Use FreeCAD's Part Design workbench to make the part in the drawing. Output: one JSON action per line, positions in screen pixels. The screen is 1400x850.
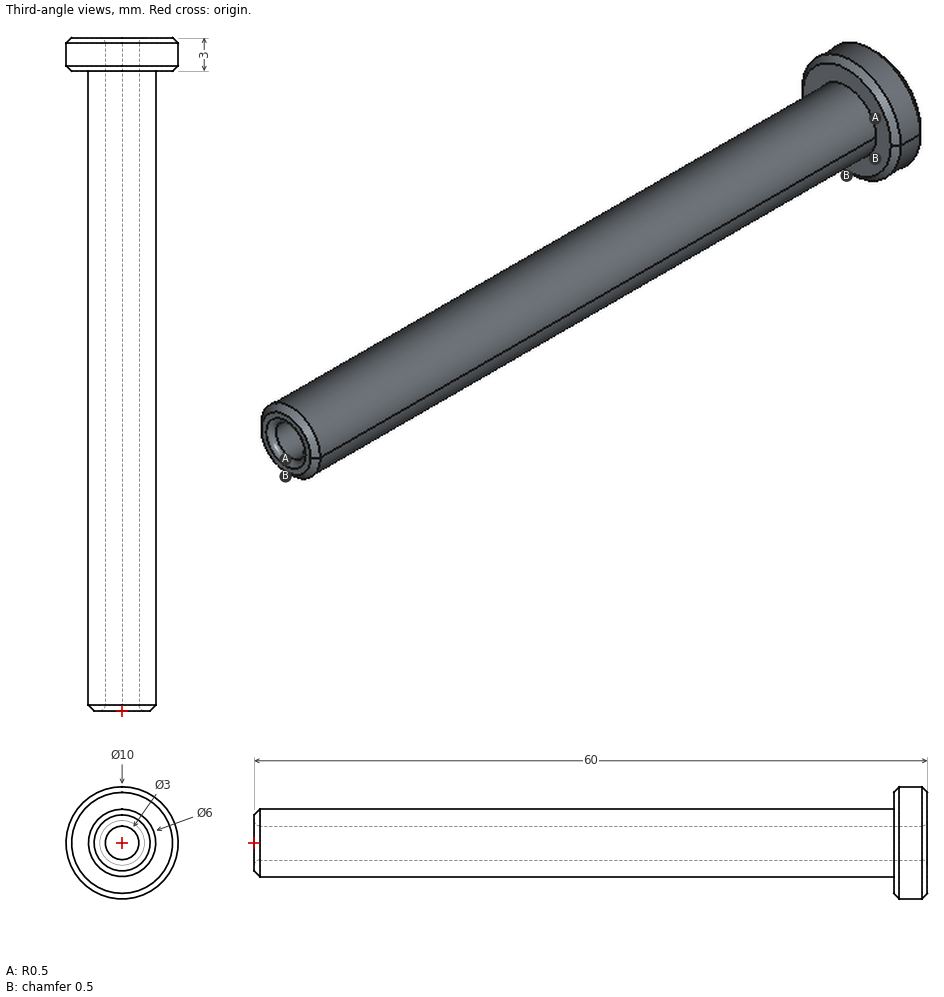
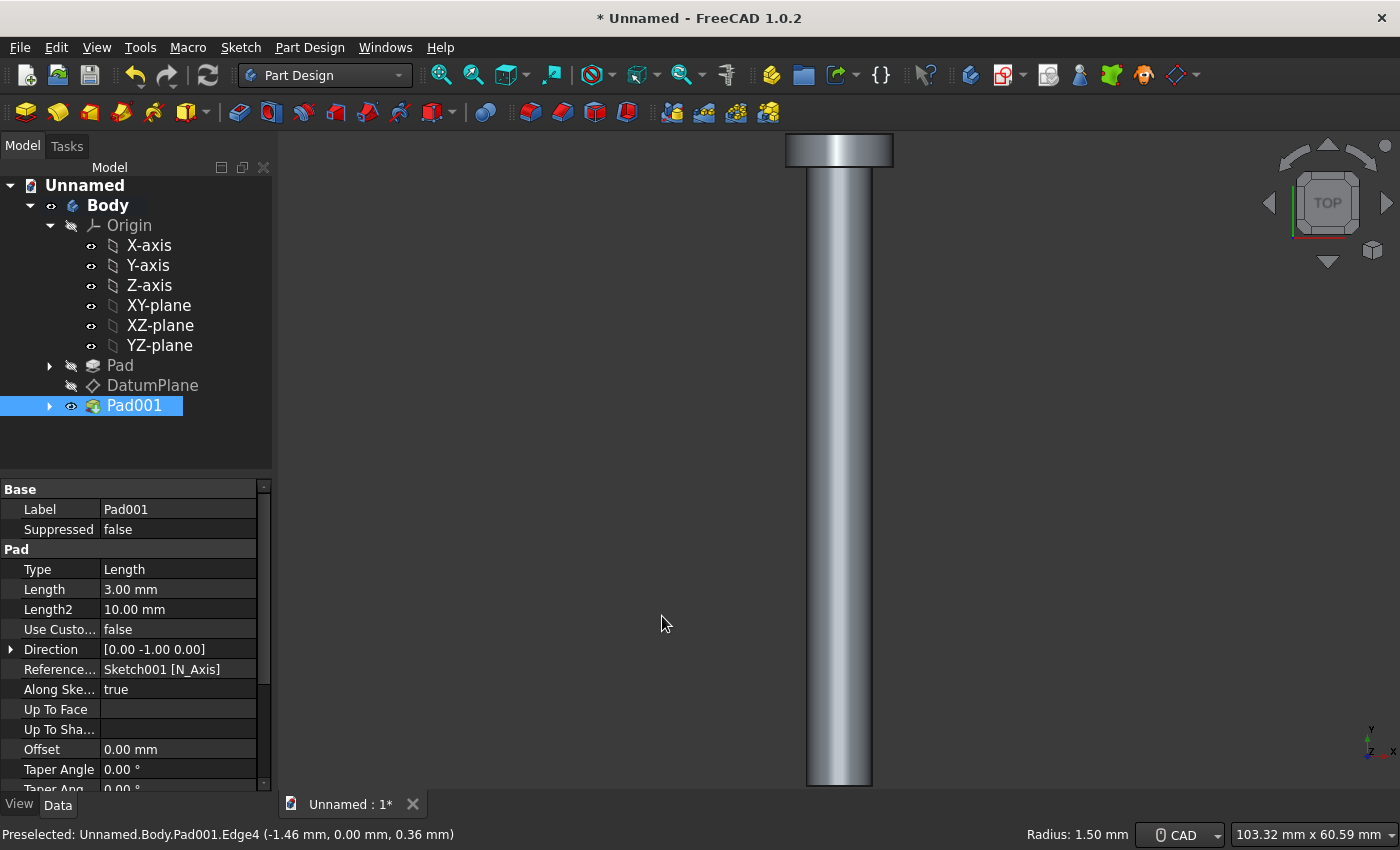
{"action": "key", "text": "1"}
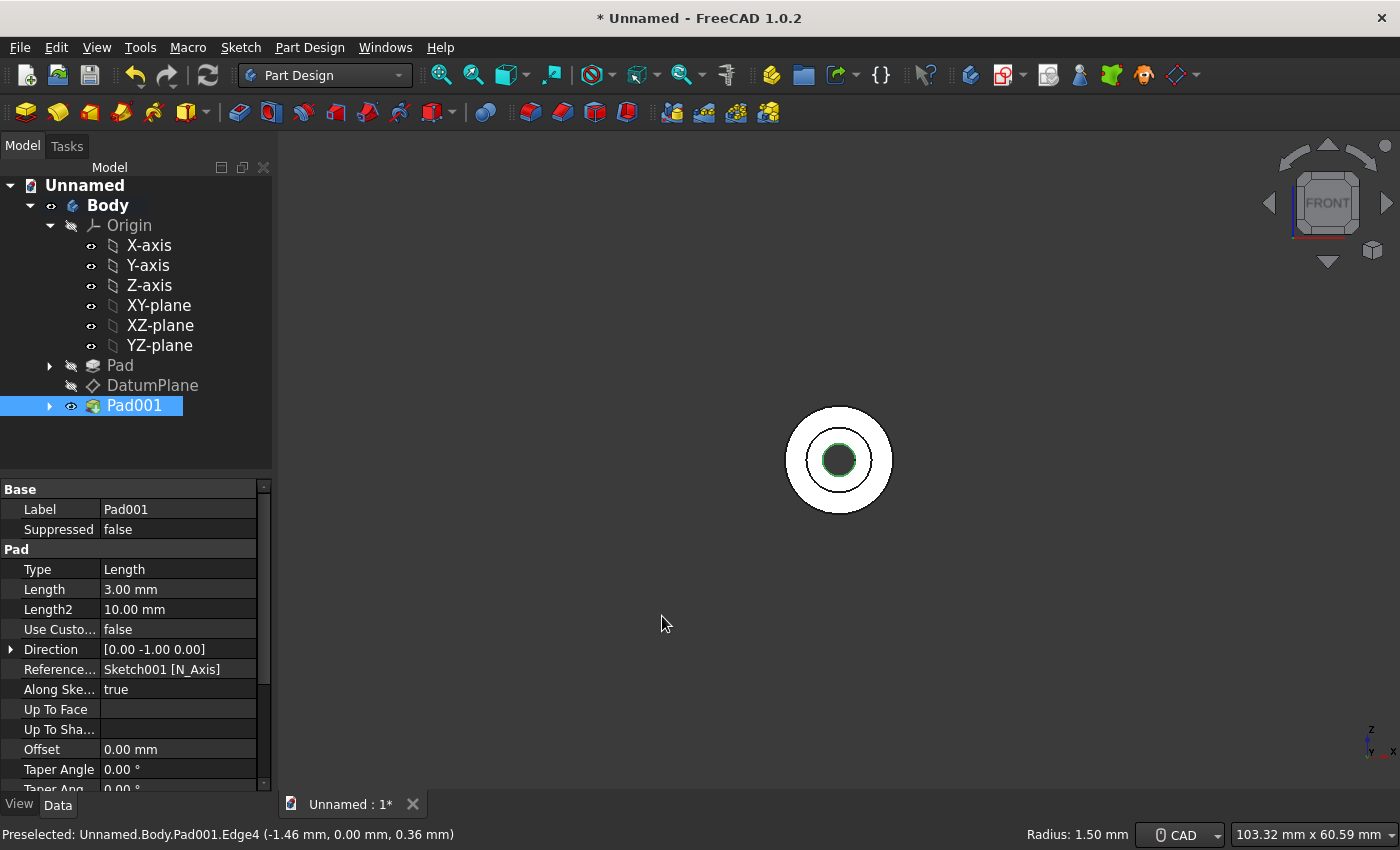
{"action": "key", "text": "v f"}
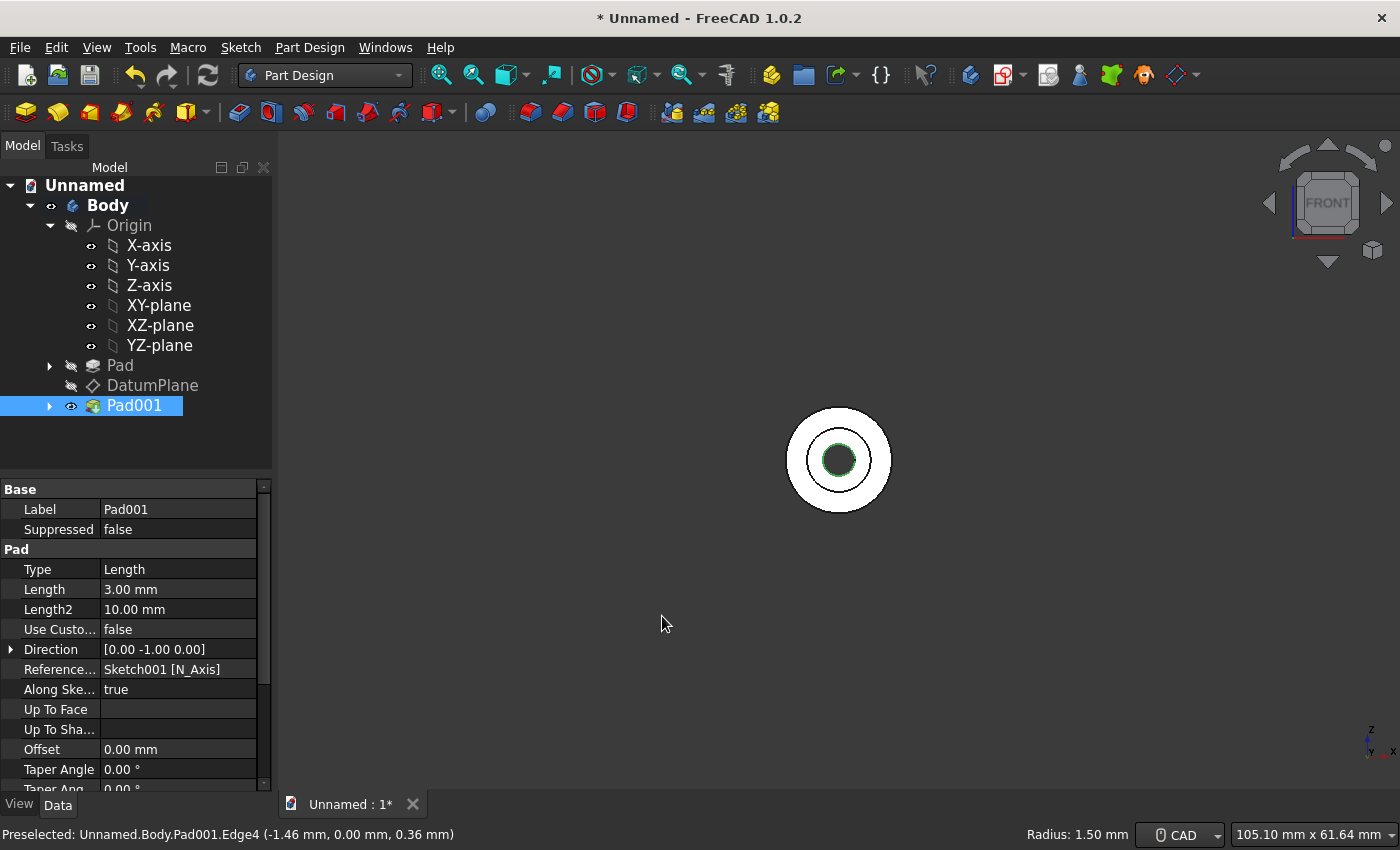
{"action": "key", "text": "3"}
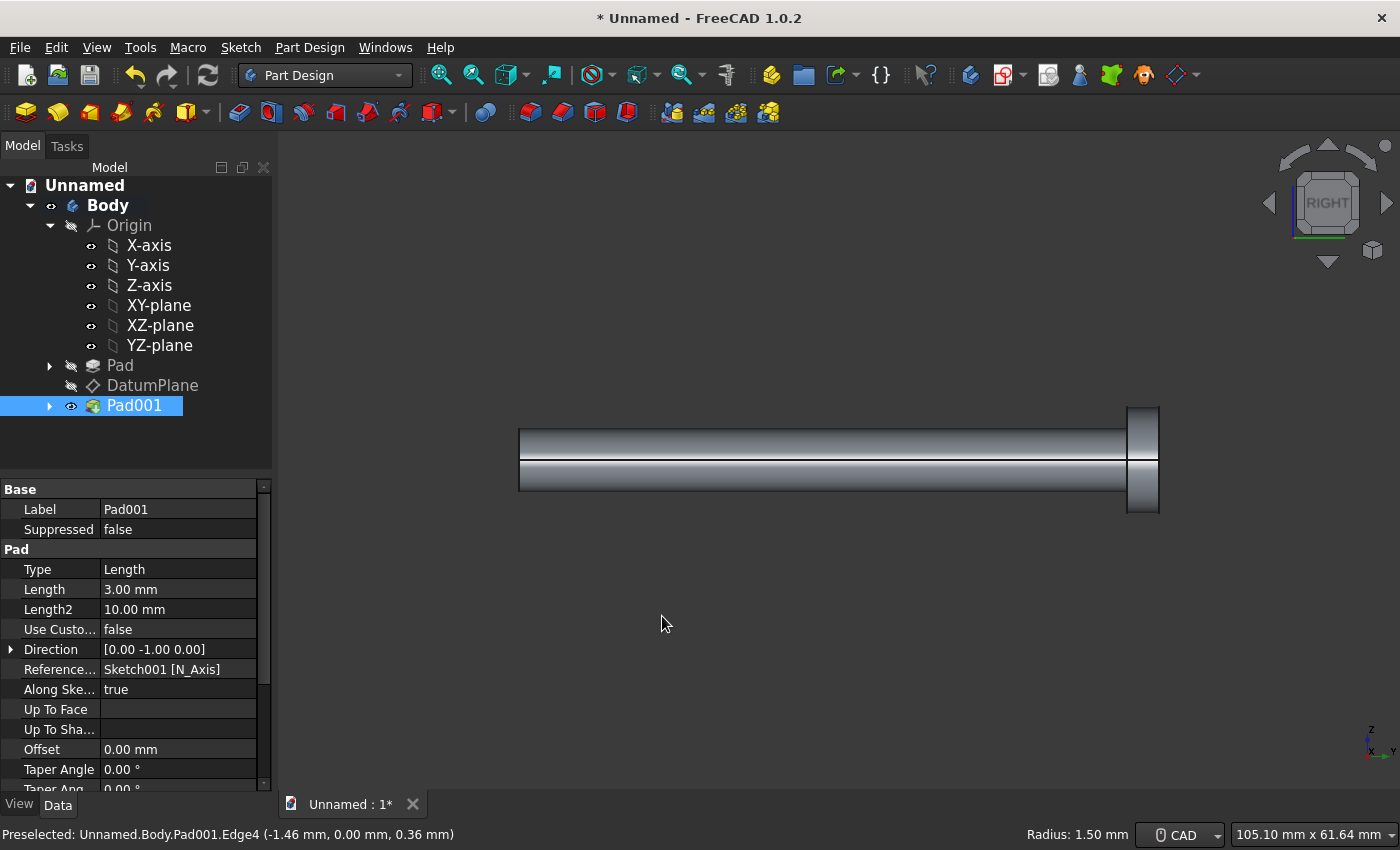
{"action": "key", "text": "5"}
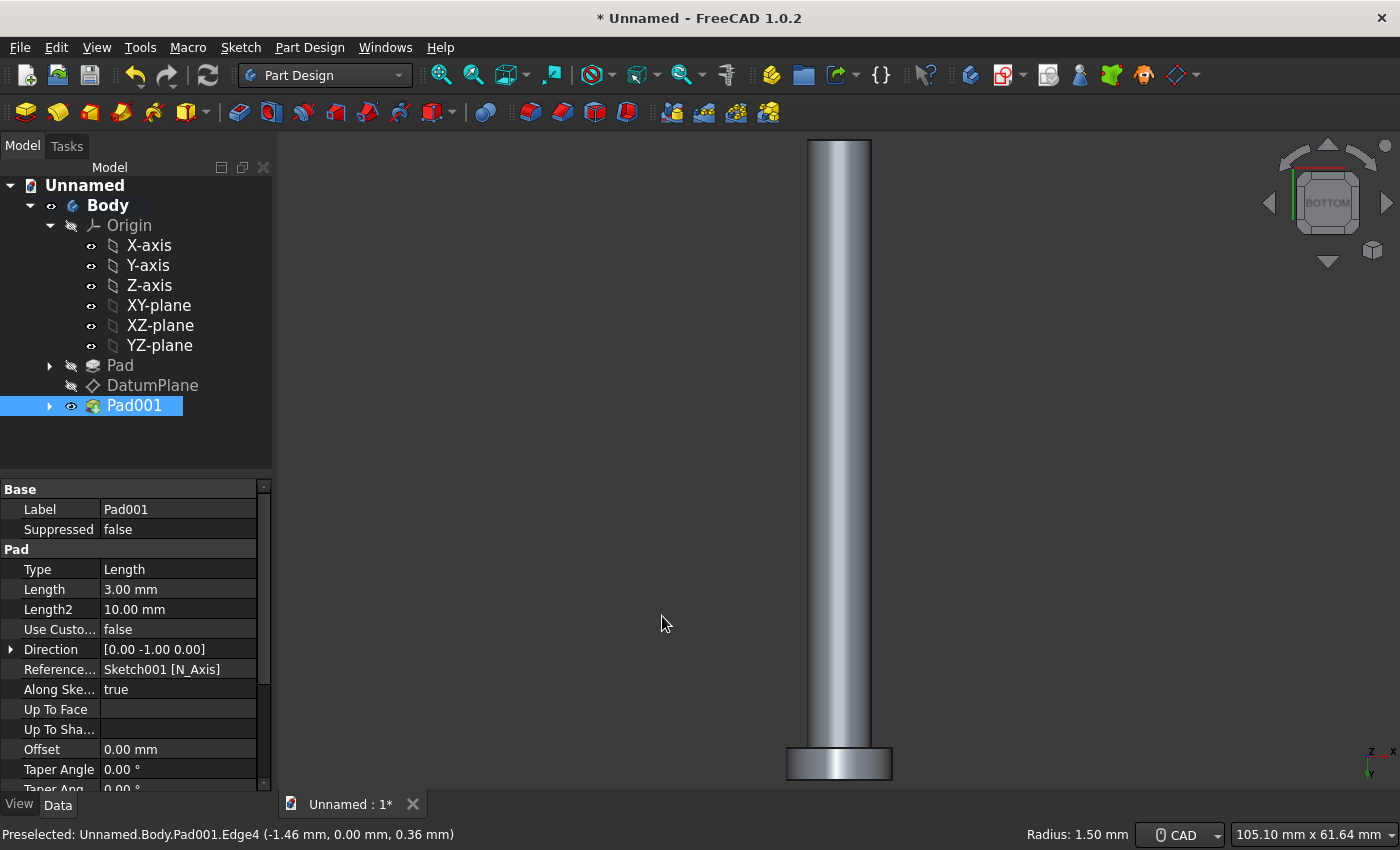
{"action": "key", "text": "4"}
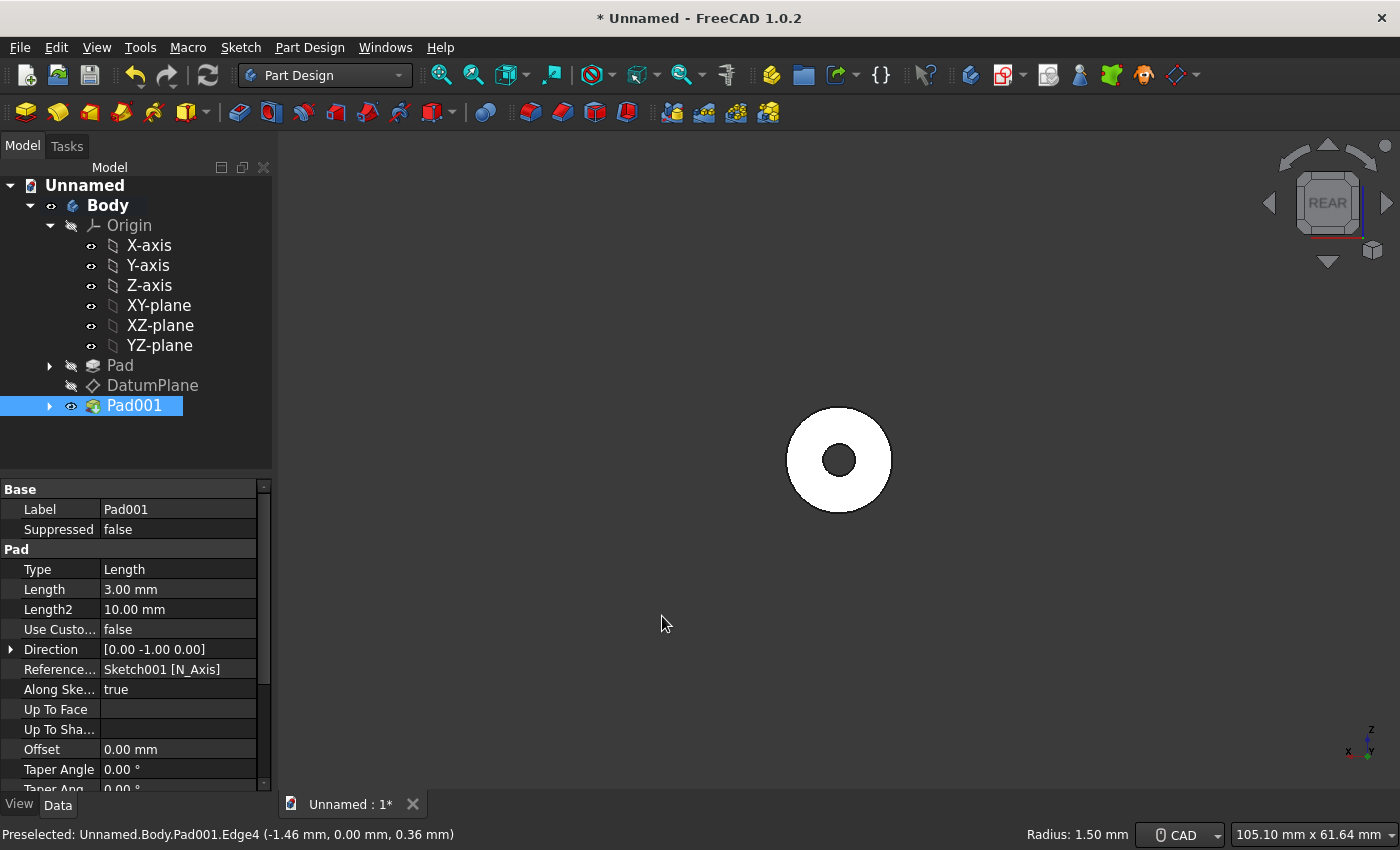
{"action": "left_click", "coordinate": [442, 76]}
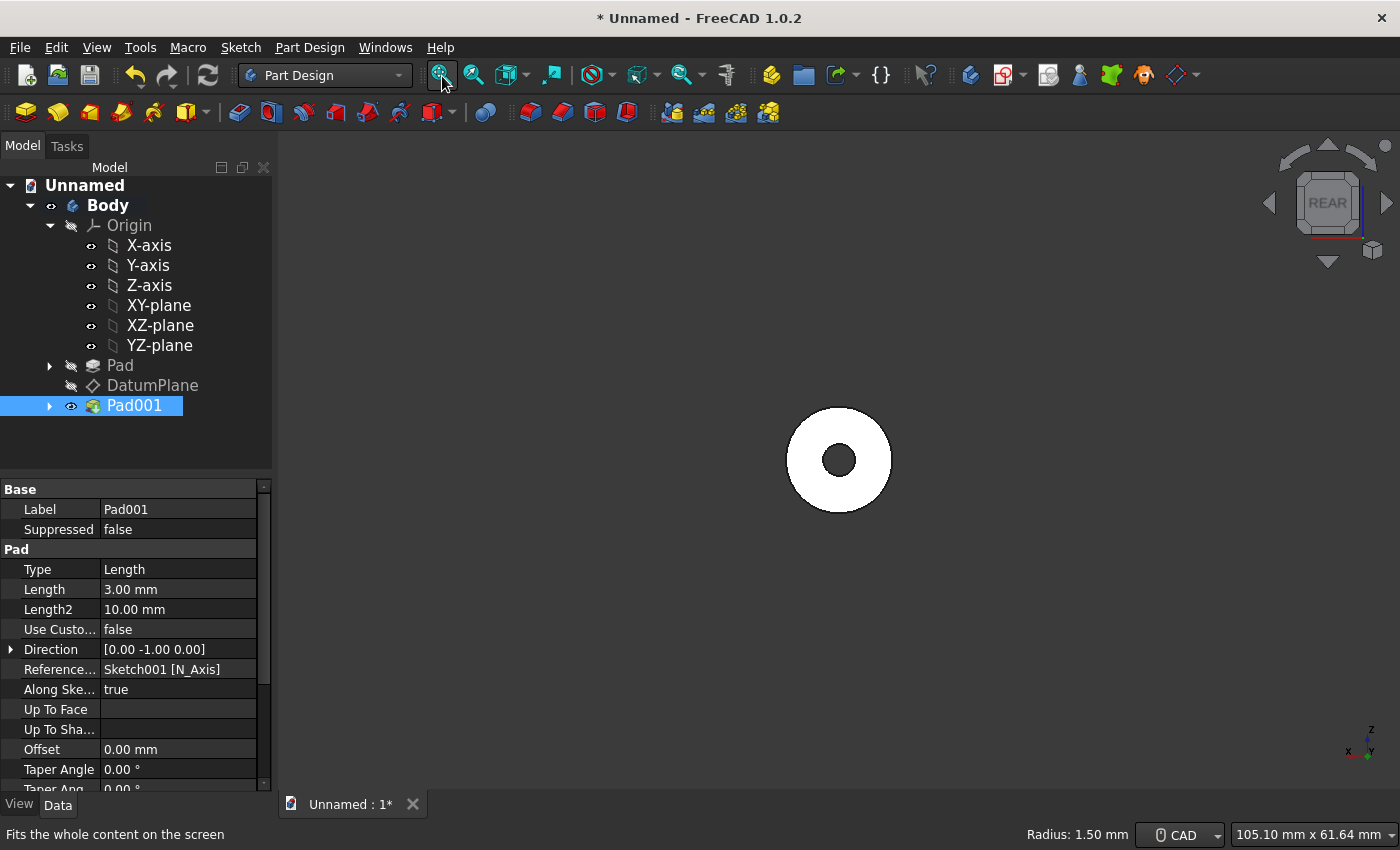
{"action": "left_click", "coordinate": [855, 459], "text": "ctrl"}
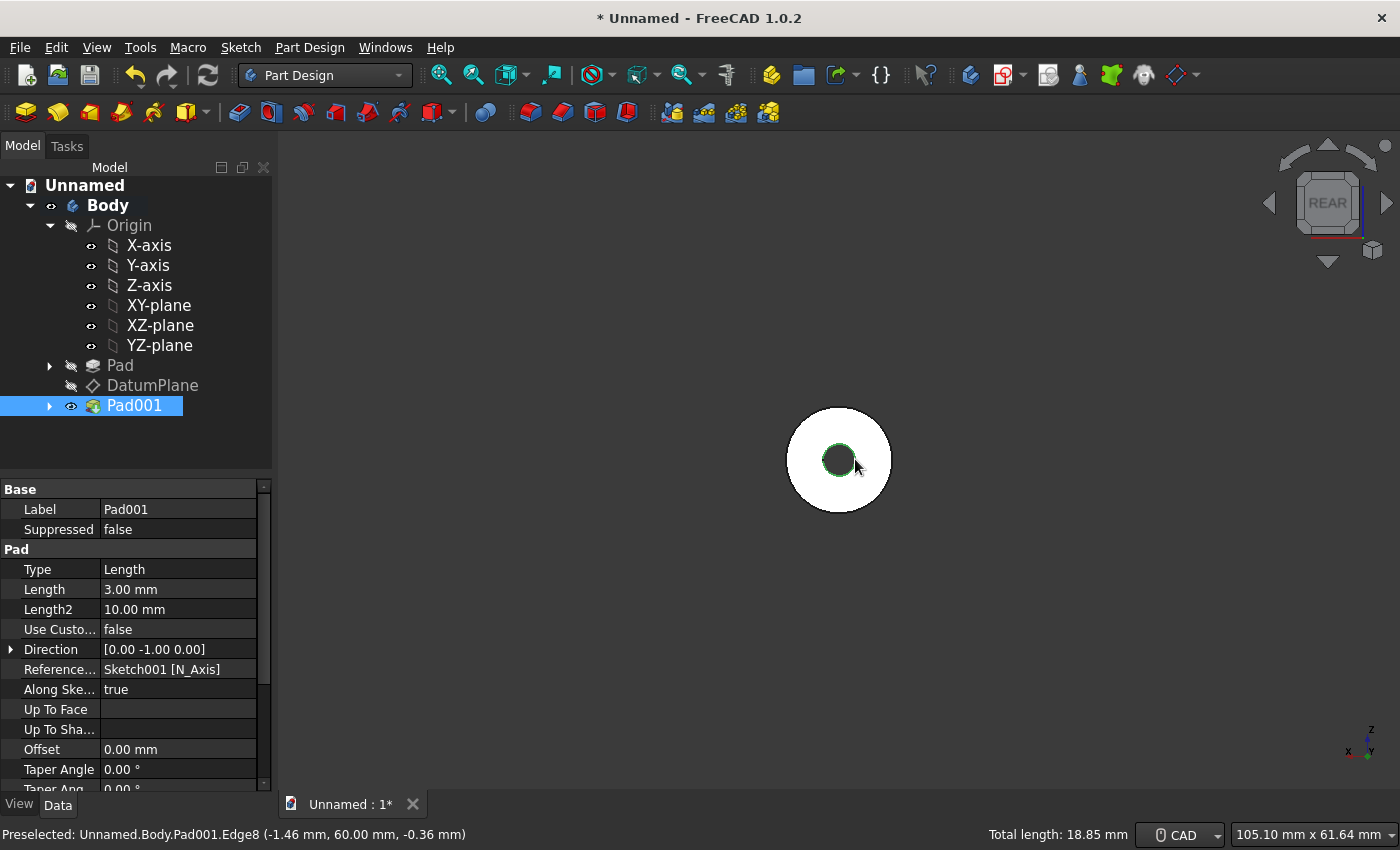
{"action": "left_click", "coordinate": [532, 112]}